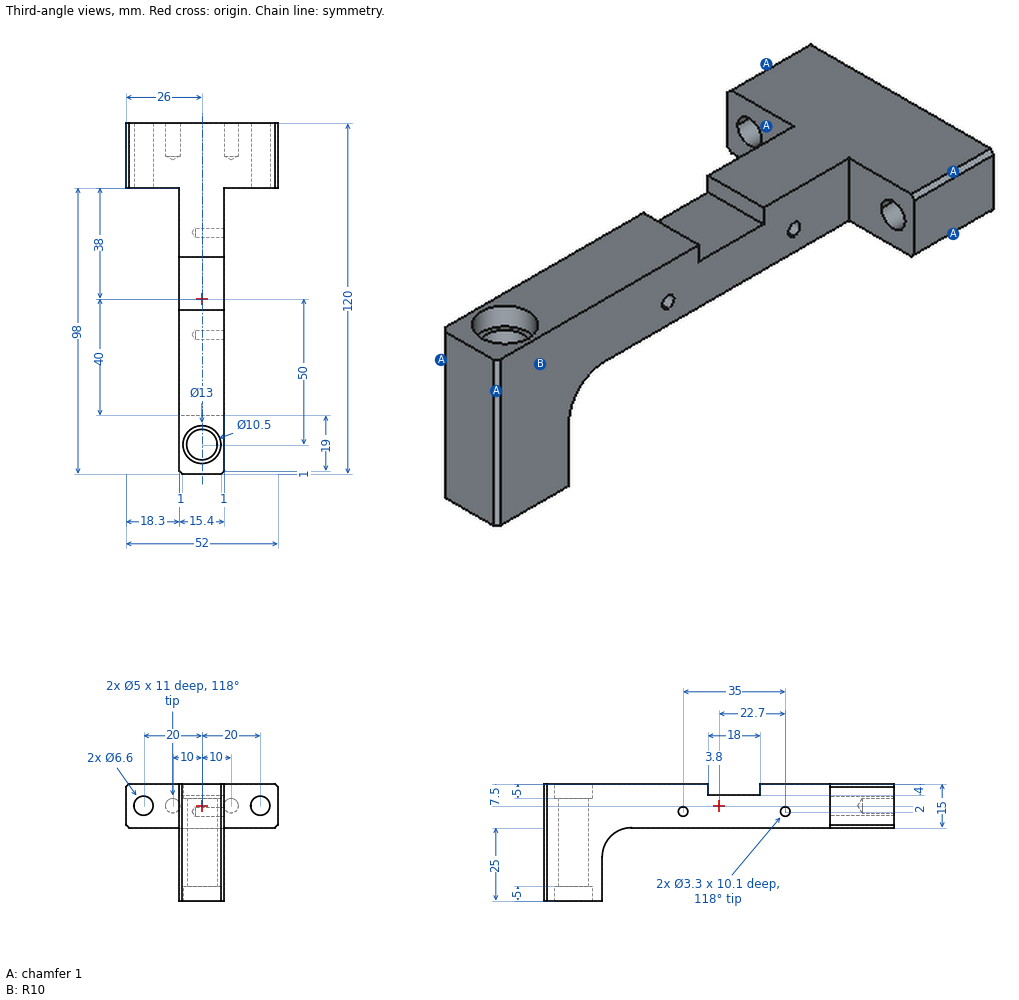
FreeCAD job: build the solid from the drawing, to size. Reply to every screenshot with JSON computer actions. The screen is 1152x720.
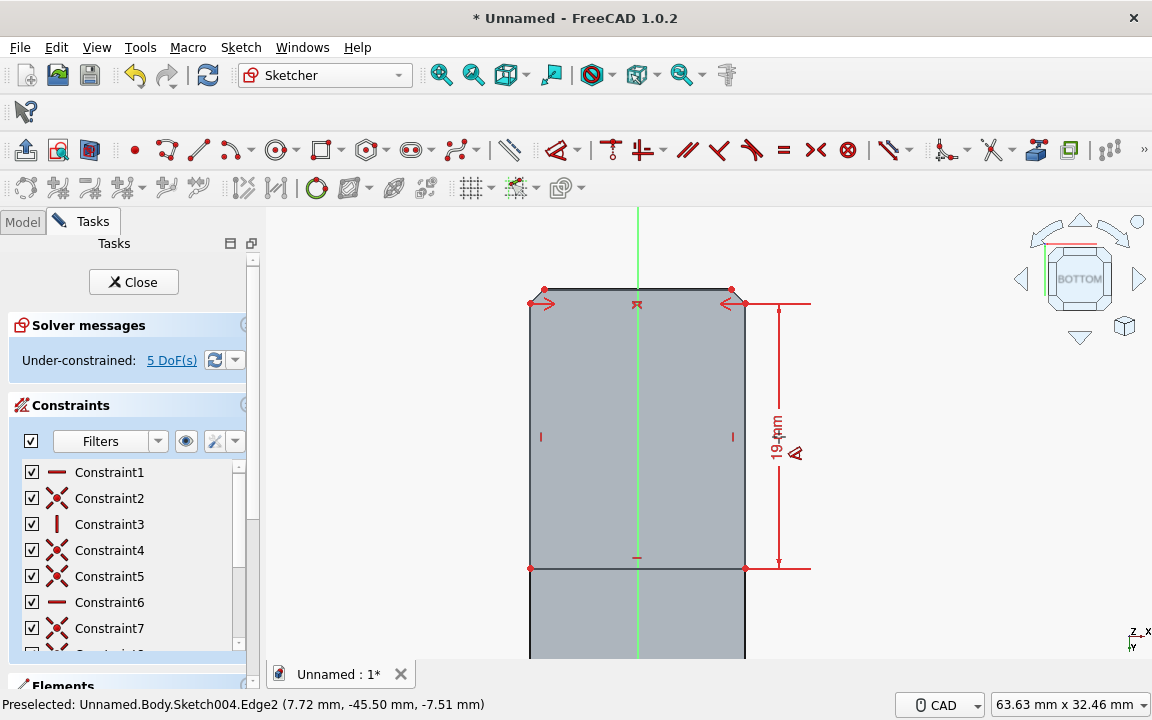
{"action": "scroll", "coordinate": [738, 297], "scroll_direction": "up", "scroll_amount": 6}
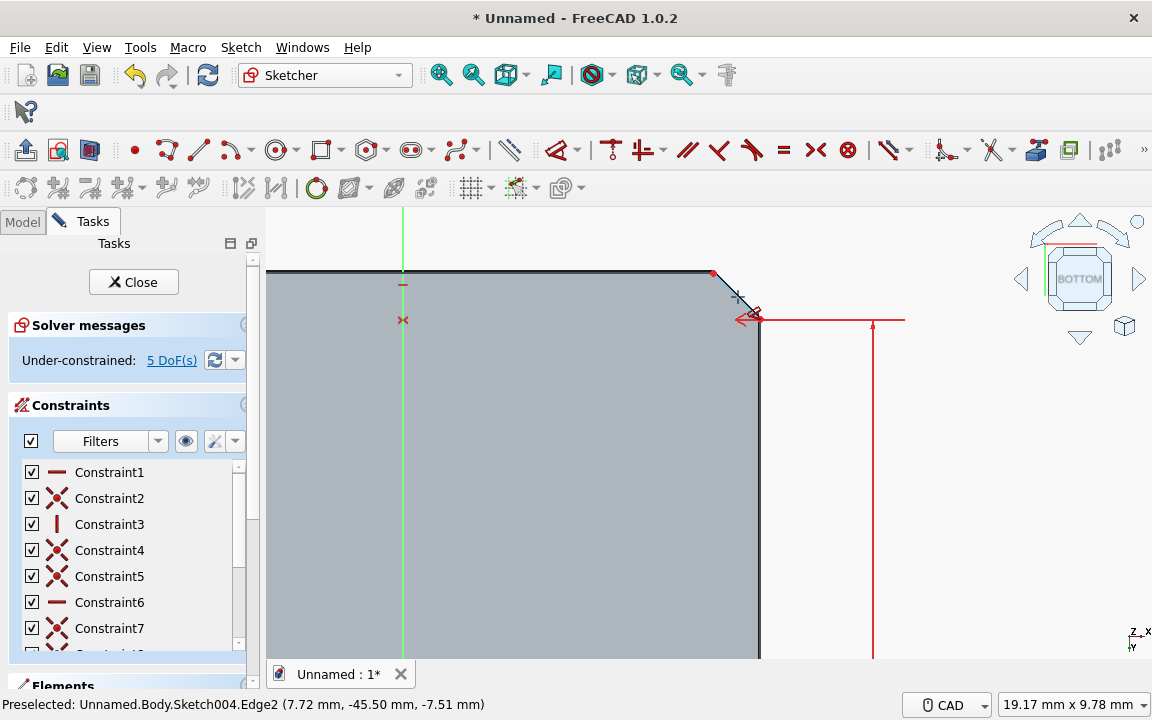
{"action": "left_click", "coordinate": [737, 297]}
{"action": "left_click", "coordinate": [737, 239]}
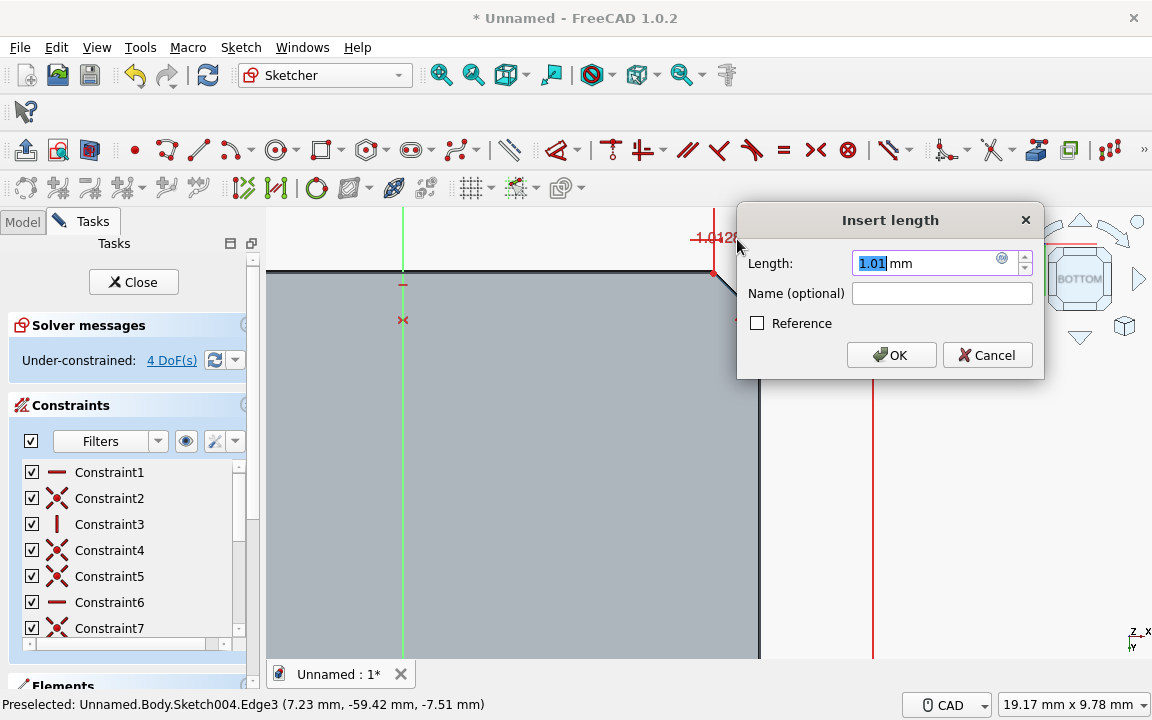
{"action": "type", "text": "1"}
{"action": "key", "text": "Return"}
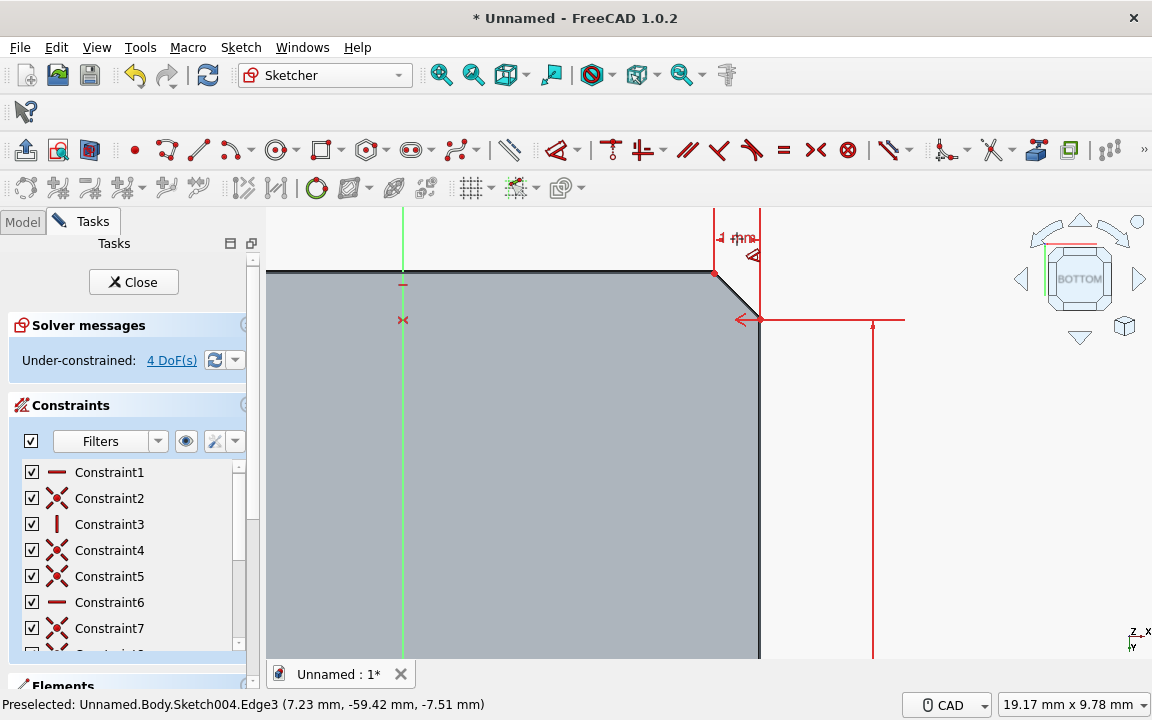
{"action": "left_click", "coordinate": [746, 306]}
{"action": "left_click", "coordinate": [794, 297]}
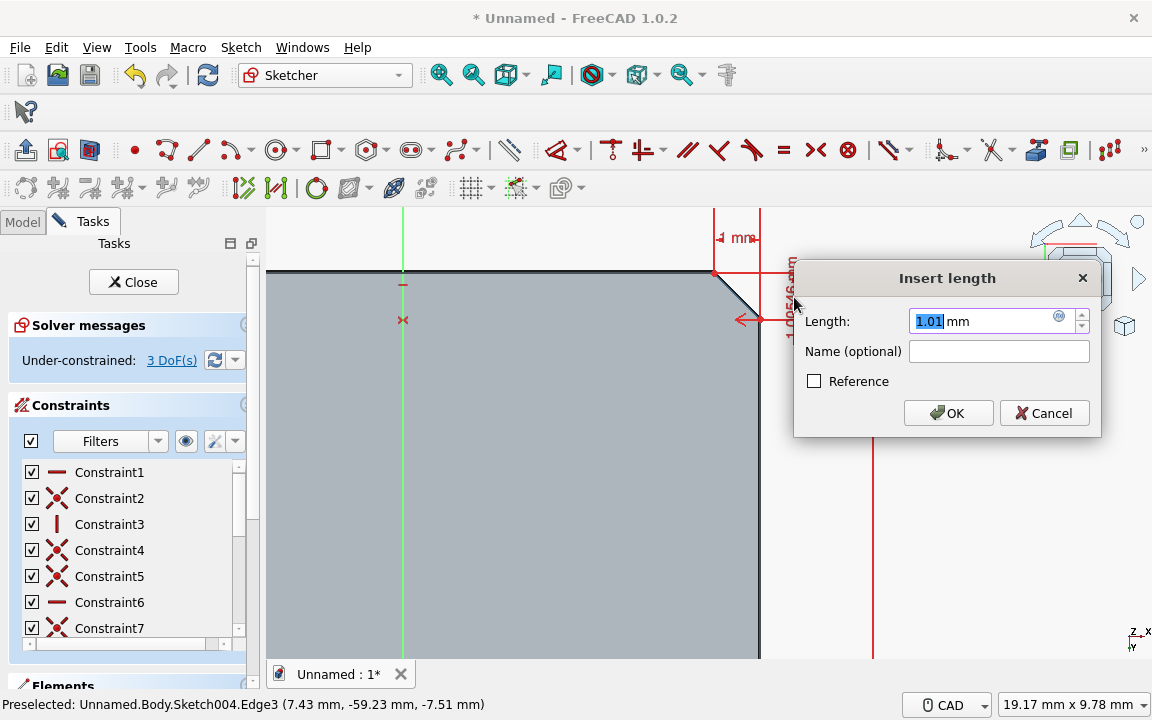
{"action": "type", "text": "1"}
{"action": "key", "text": "Return"}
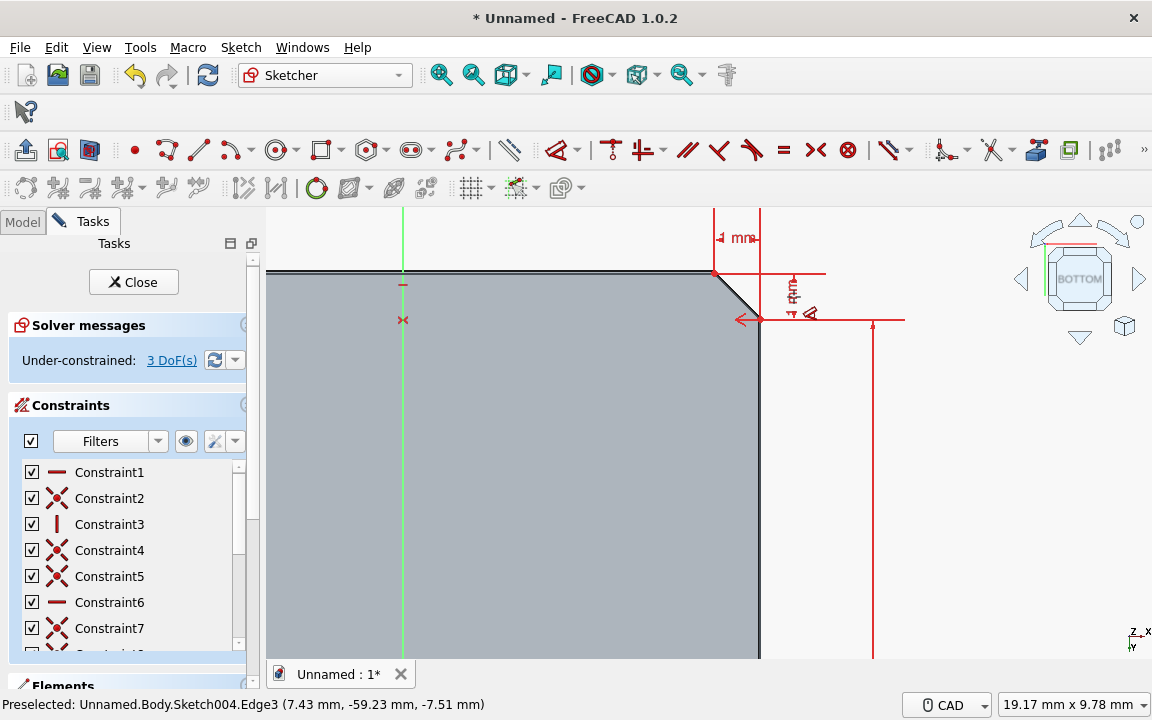
{"action": "scroll", "coordinate": [743, 304], "scroll_direction": "down", "scroll_amount": 6}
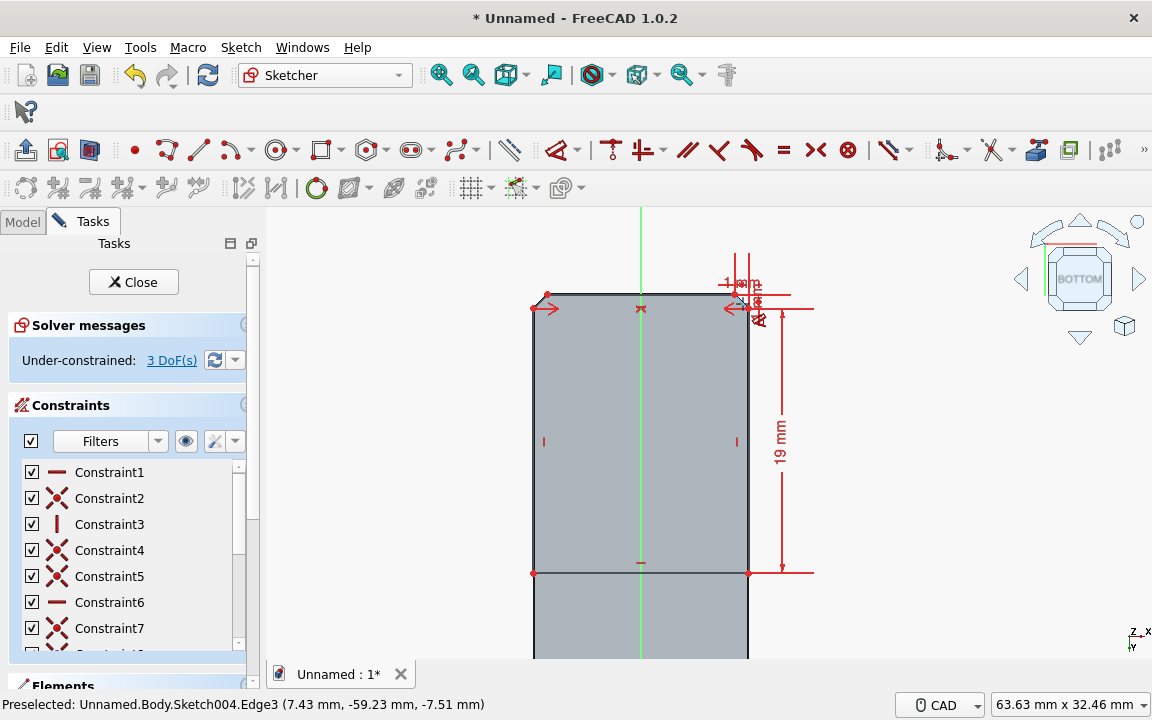
{"action": "scroll", "coordinate": [543, 299], "scroll_direction": "up", "scroll_amount": 6}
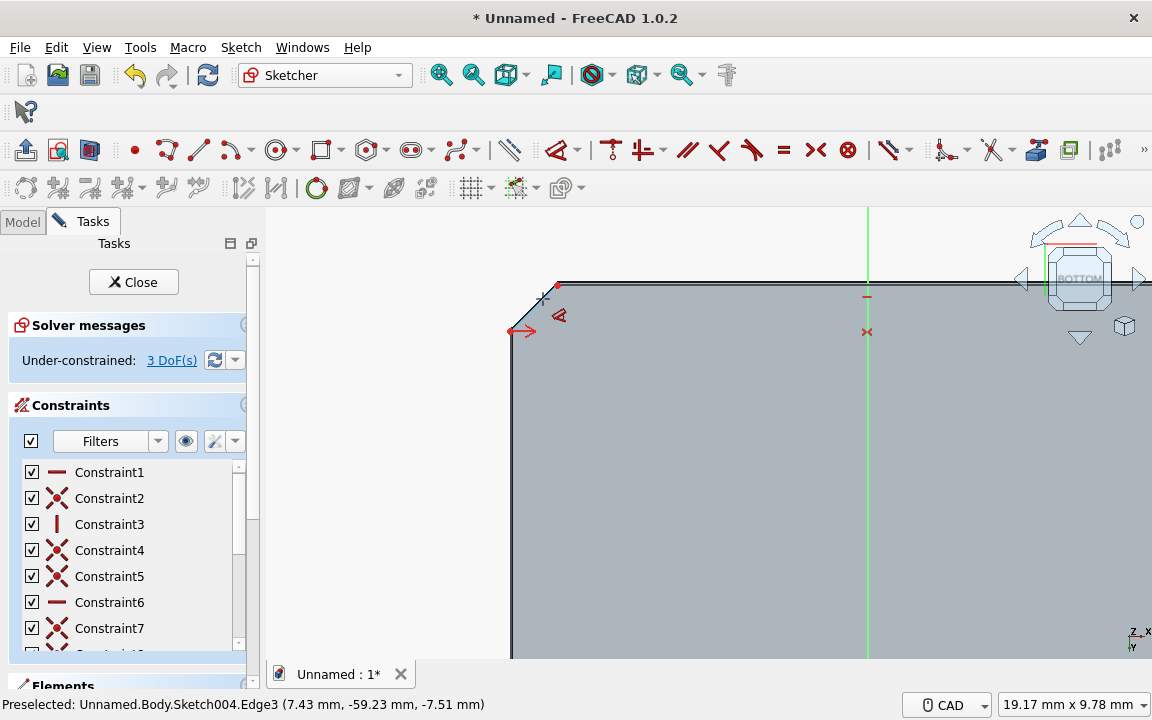
{"action": "left_click", "coordinate": [543, 299]}
{"action": "left_click", "coordinate": [534, 251]}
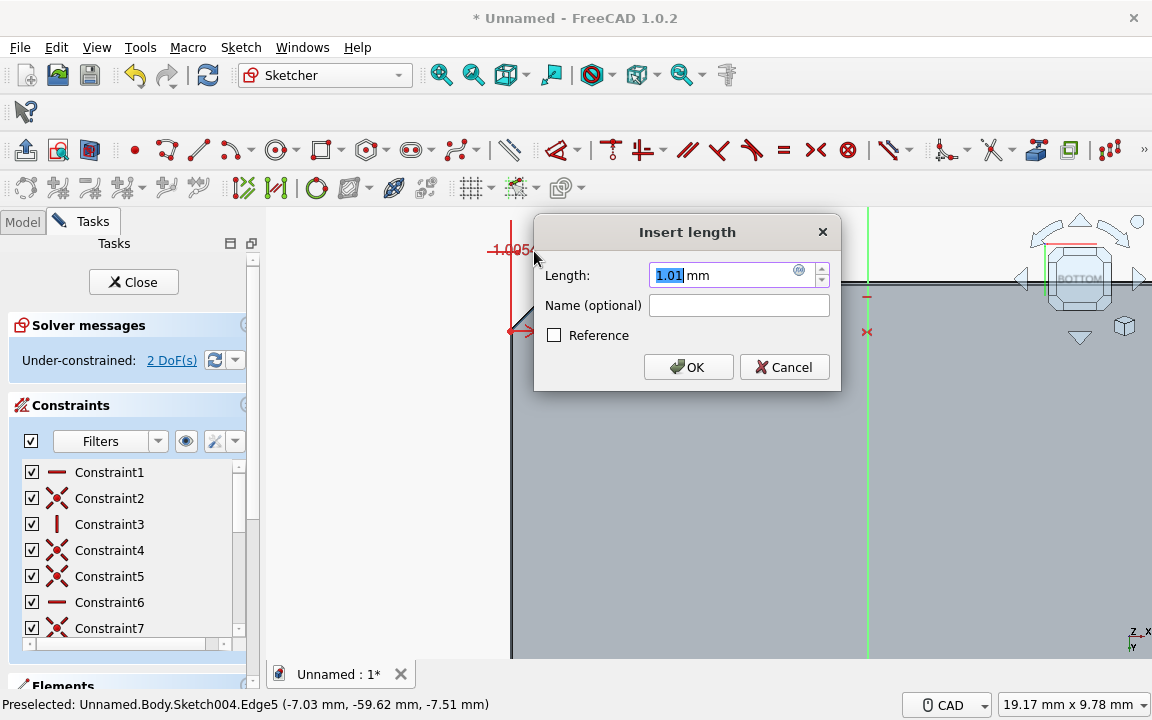
{"action": "type", "text": "1"}
{"action": "key", "text": "Return"}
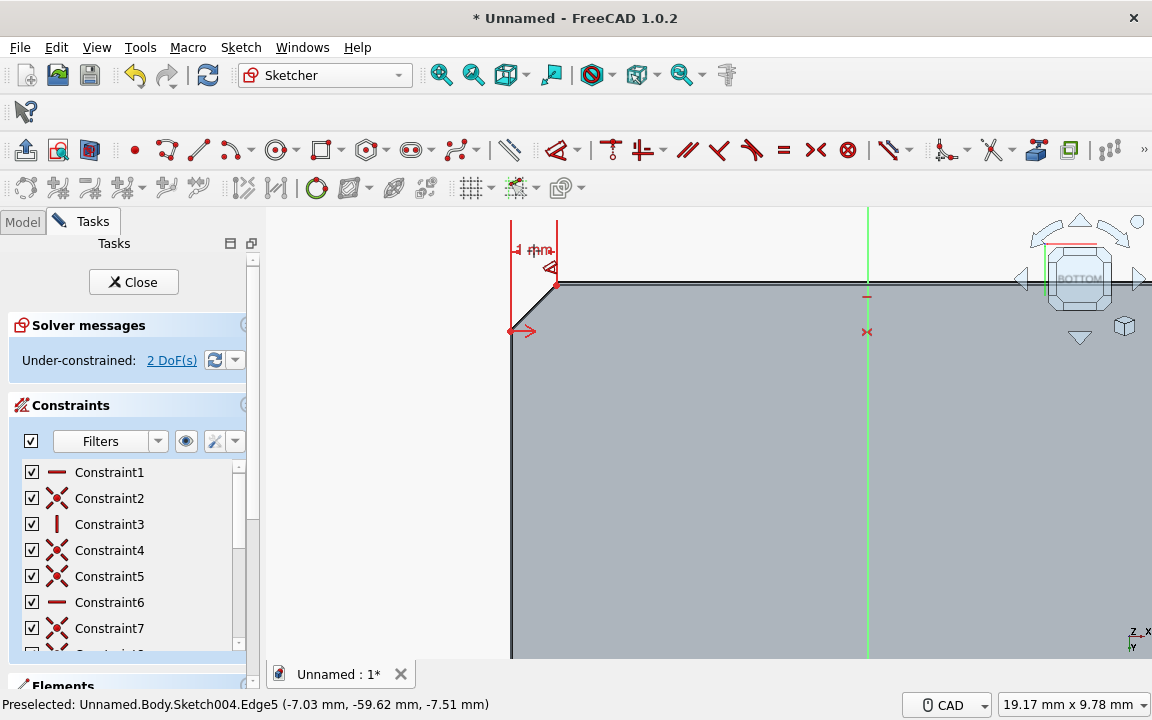
{"action": "scroll", "coordinate": [543, 299], "scroll_direction": "down", "scroll_amount": 6}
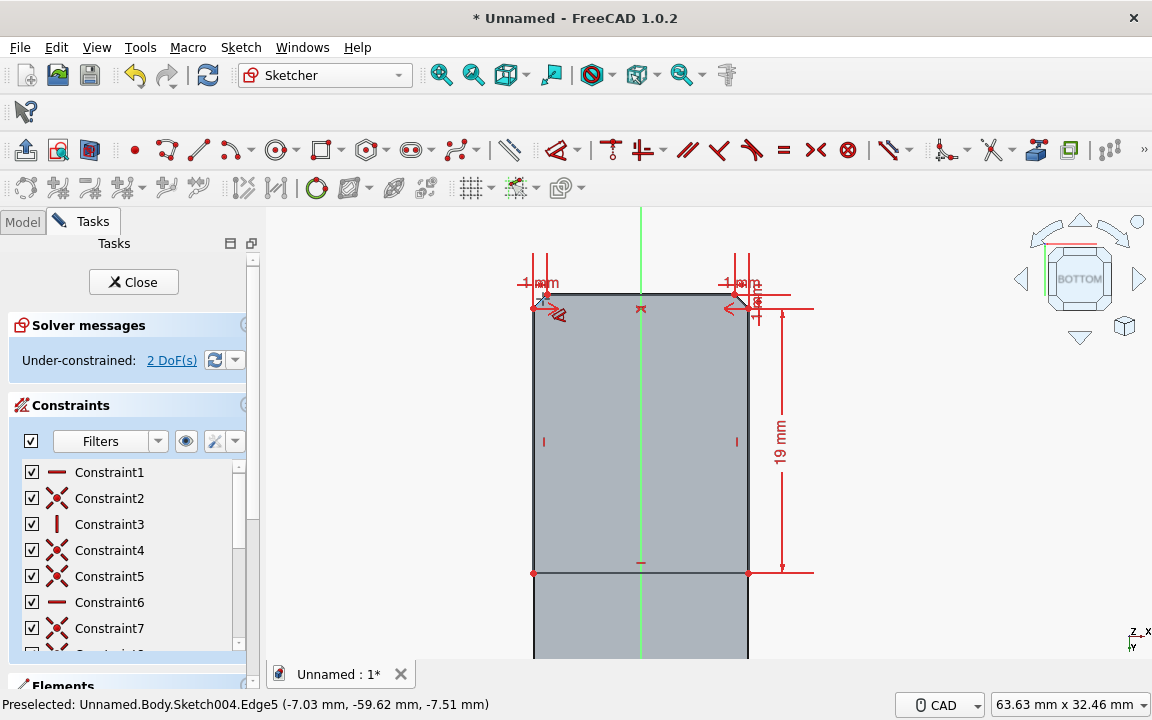
{"action": "left_click", "coordinate": [533, 573]}
{"action": "left_click", "coordinate": [499, 602]}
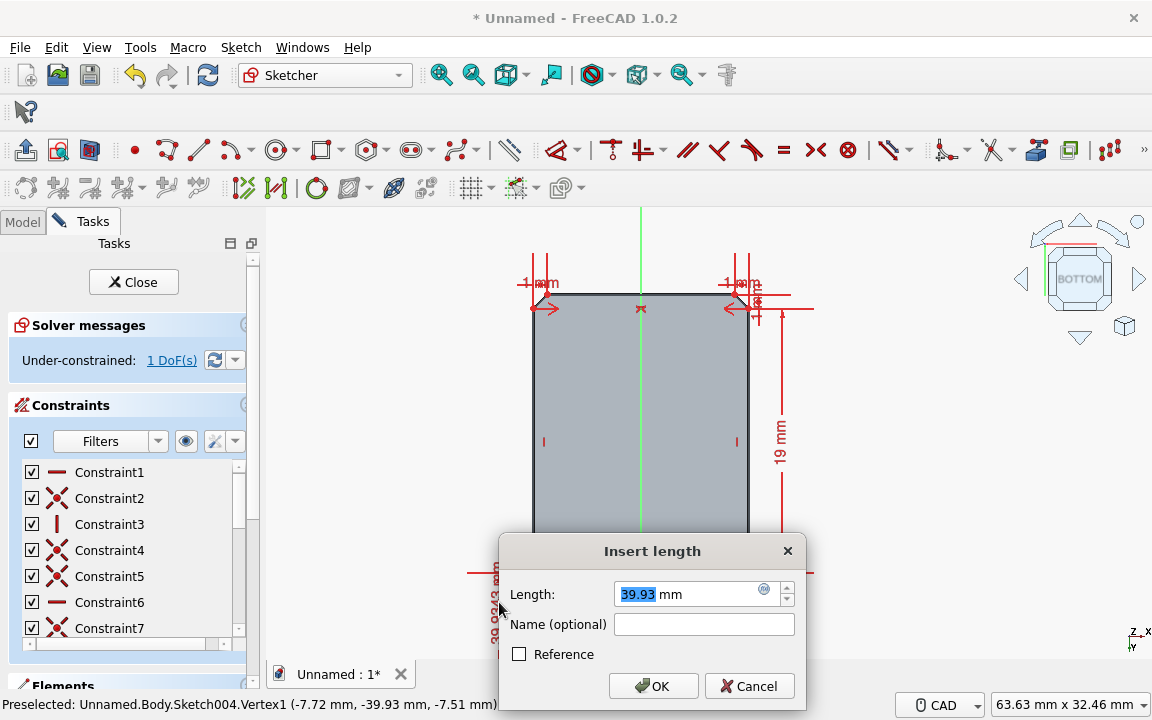
{"action": "type", "text": "40"}
{"action": "key", "text": "Return"}